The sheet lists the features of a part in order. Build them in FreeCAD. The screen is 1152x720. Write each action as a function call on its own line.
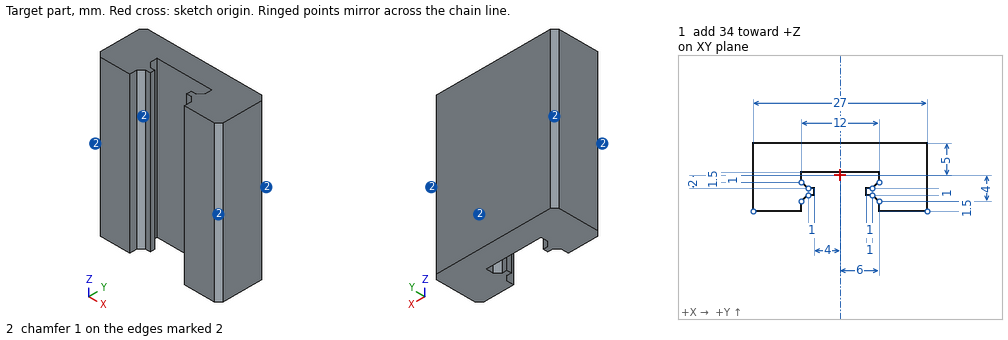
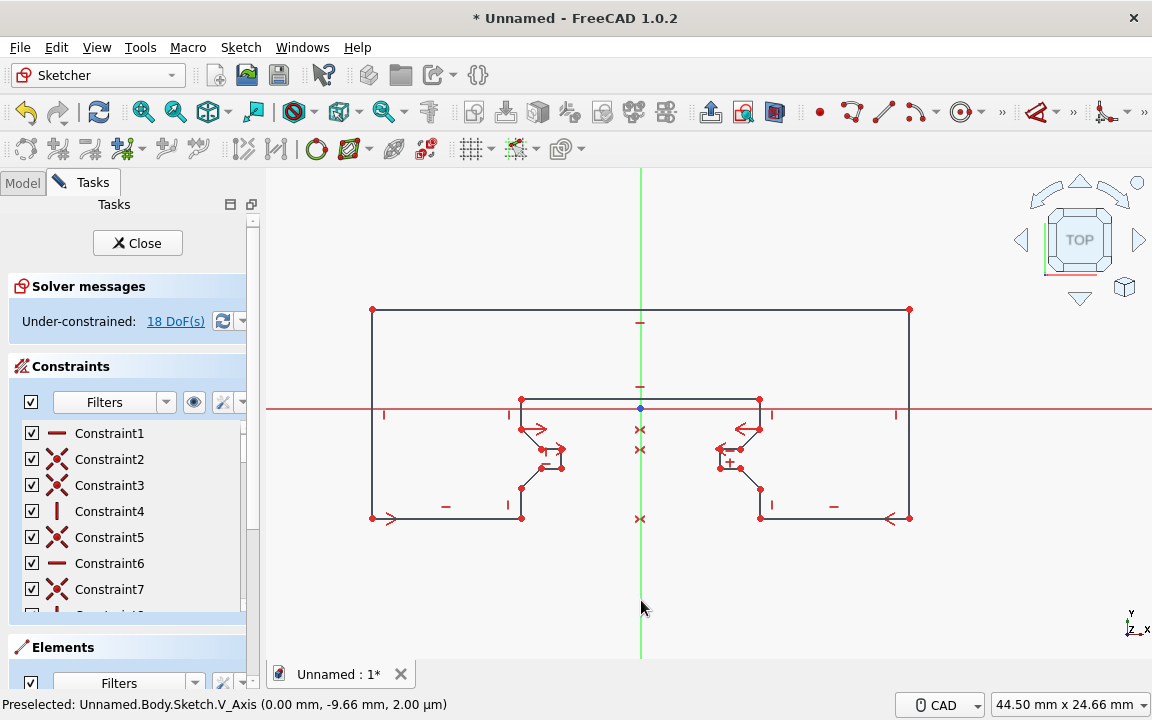
click(760, 489)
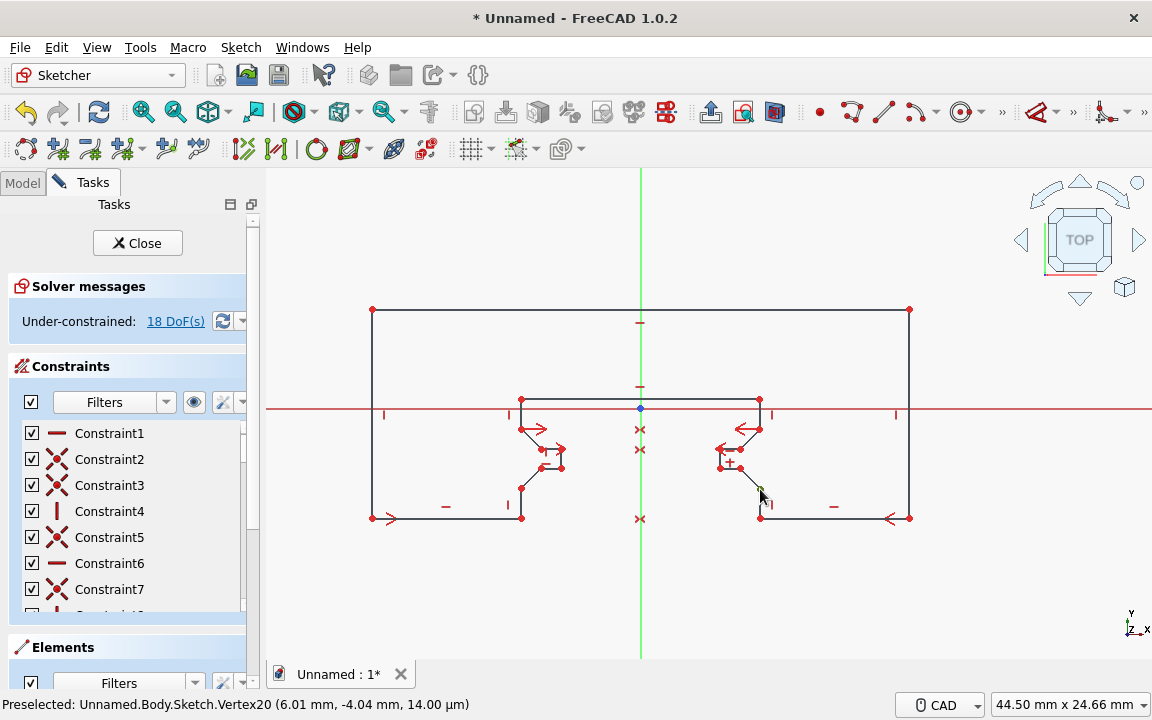
click(521, 489)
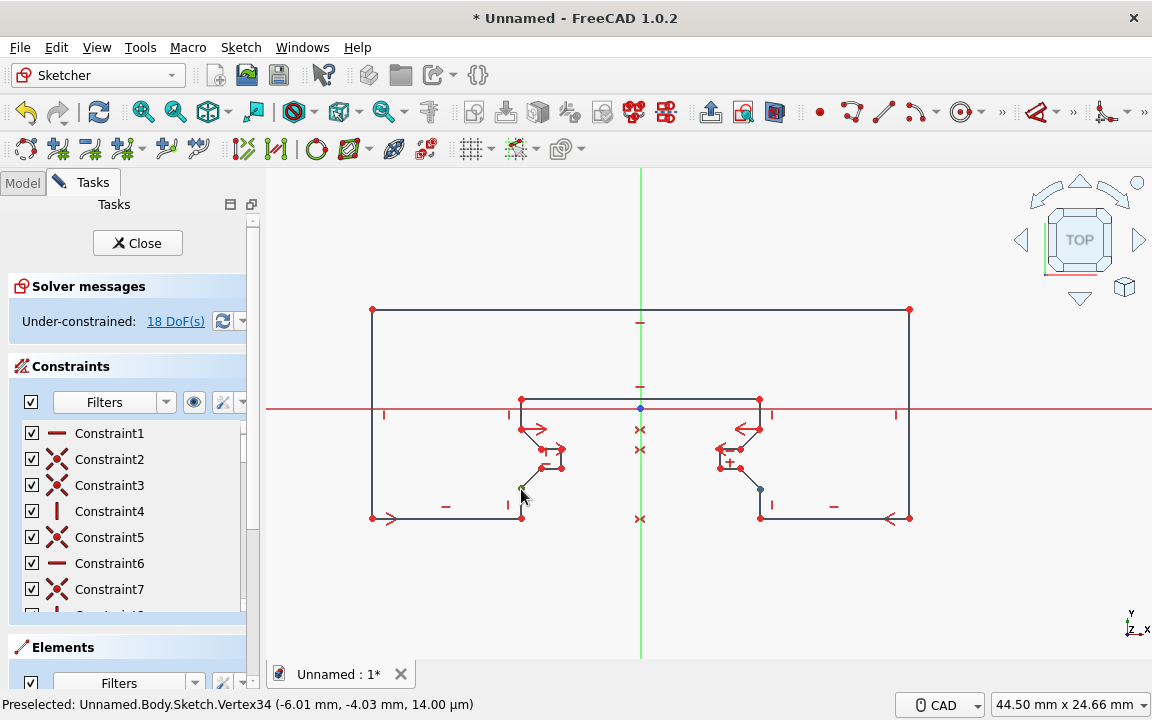
click(641, 600)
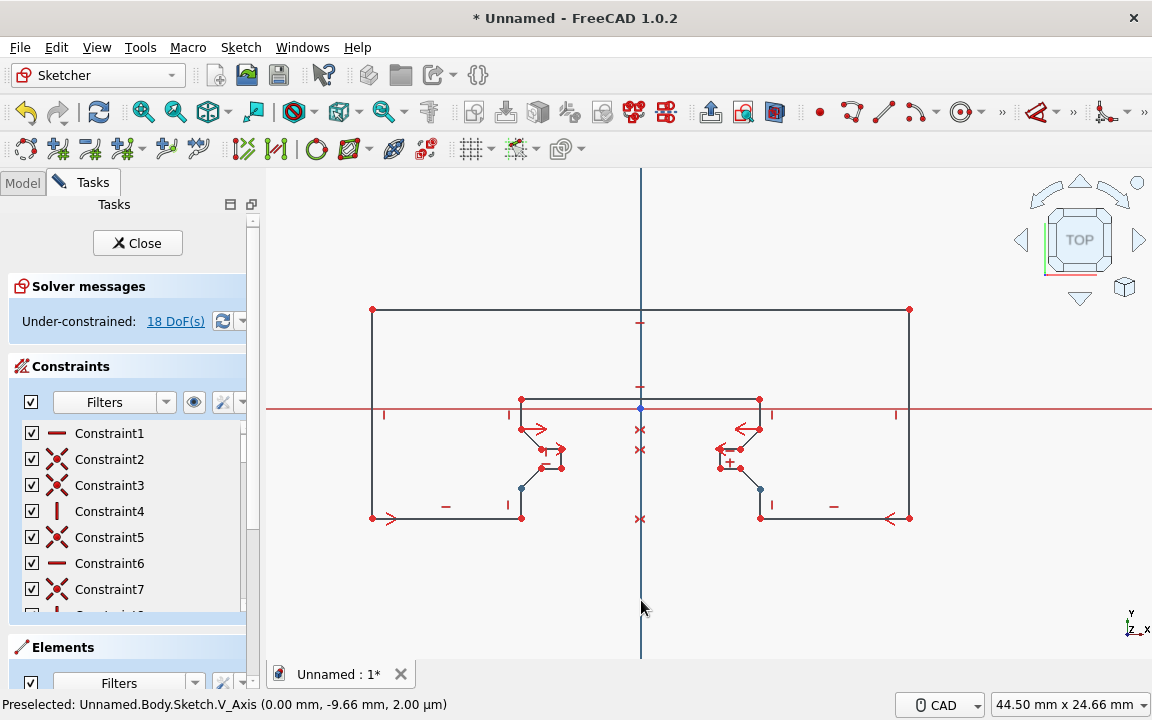
key(s)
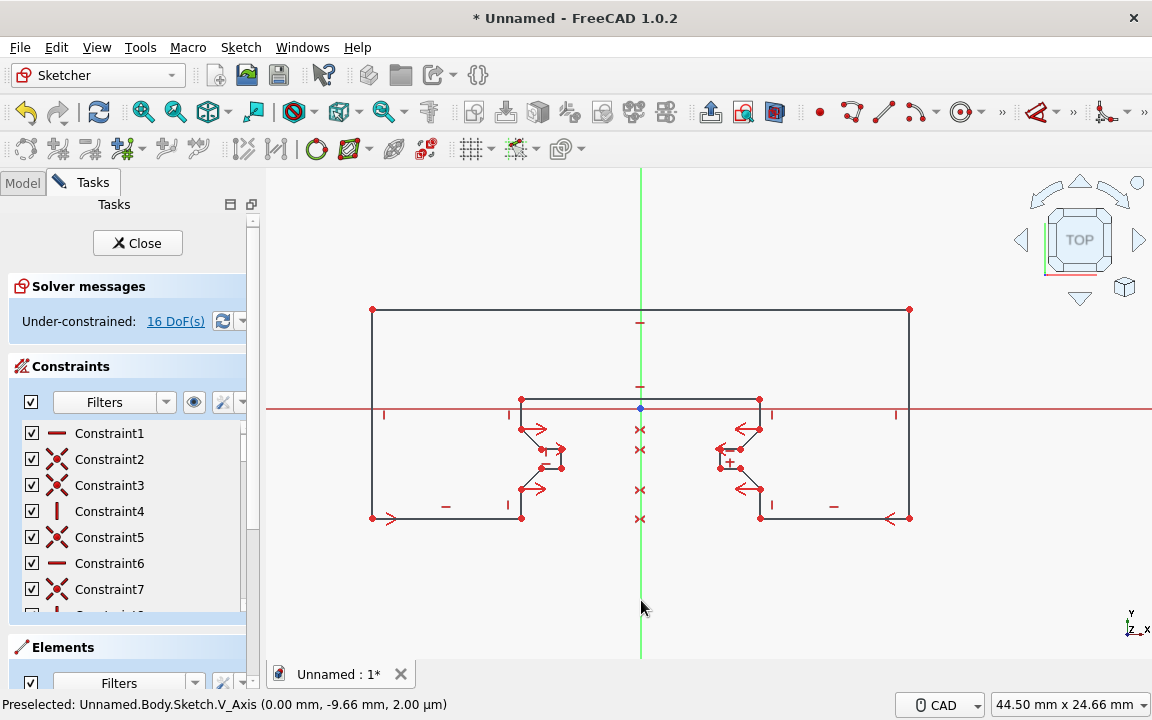
click(740, 469)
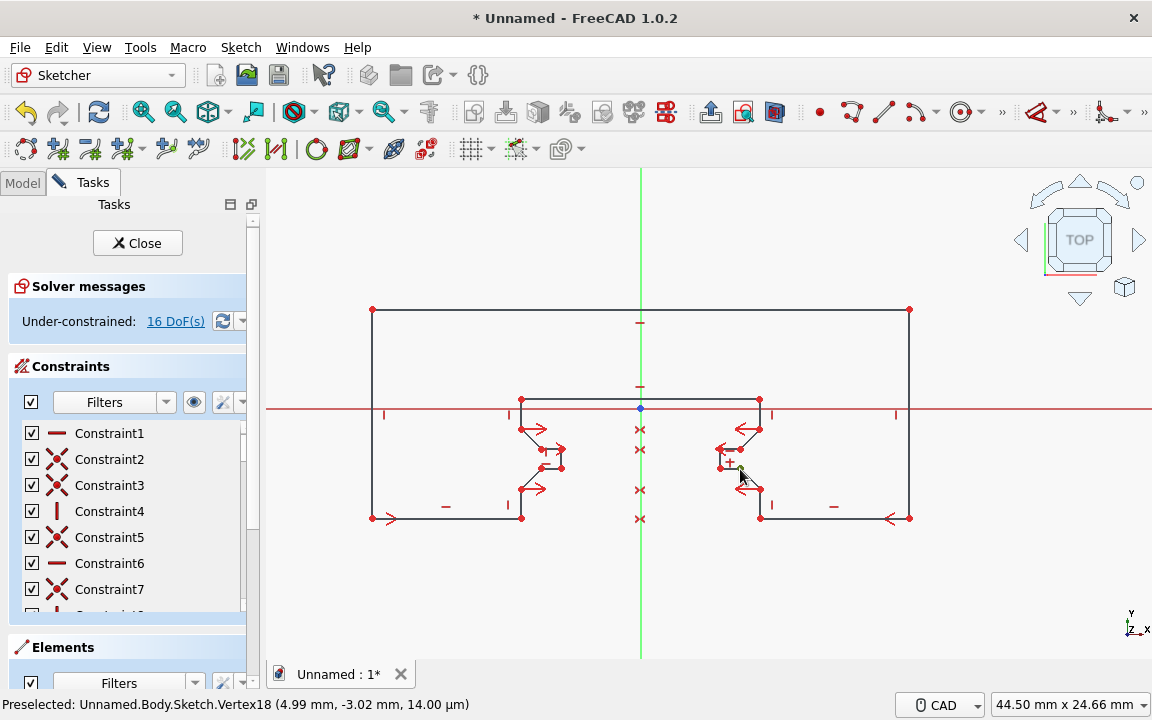
click(541, 469)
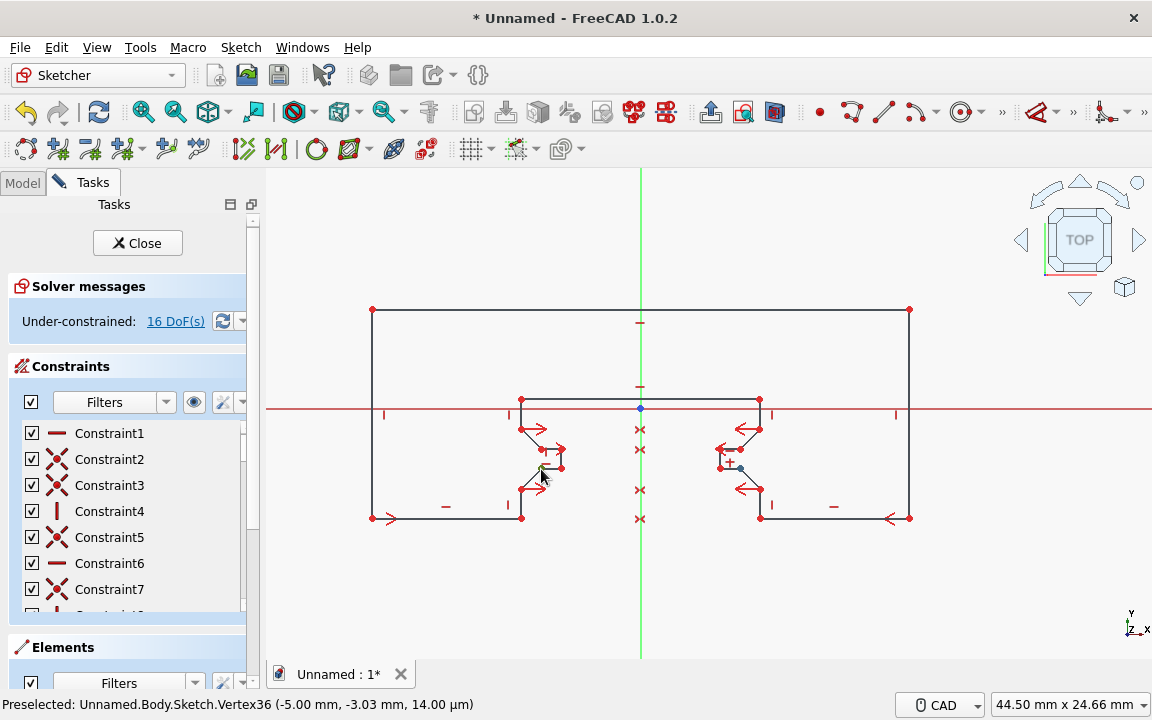
click(641, 600)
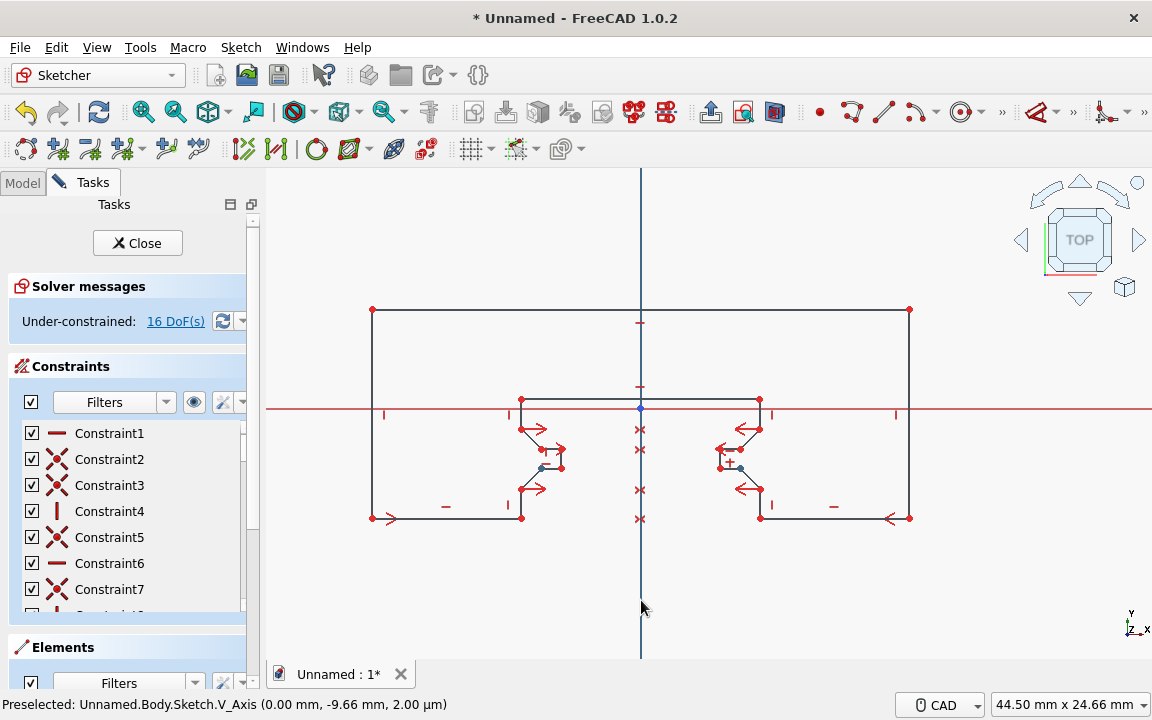
key(s)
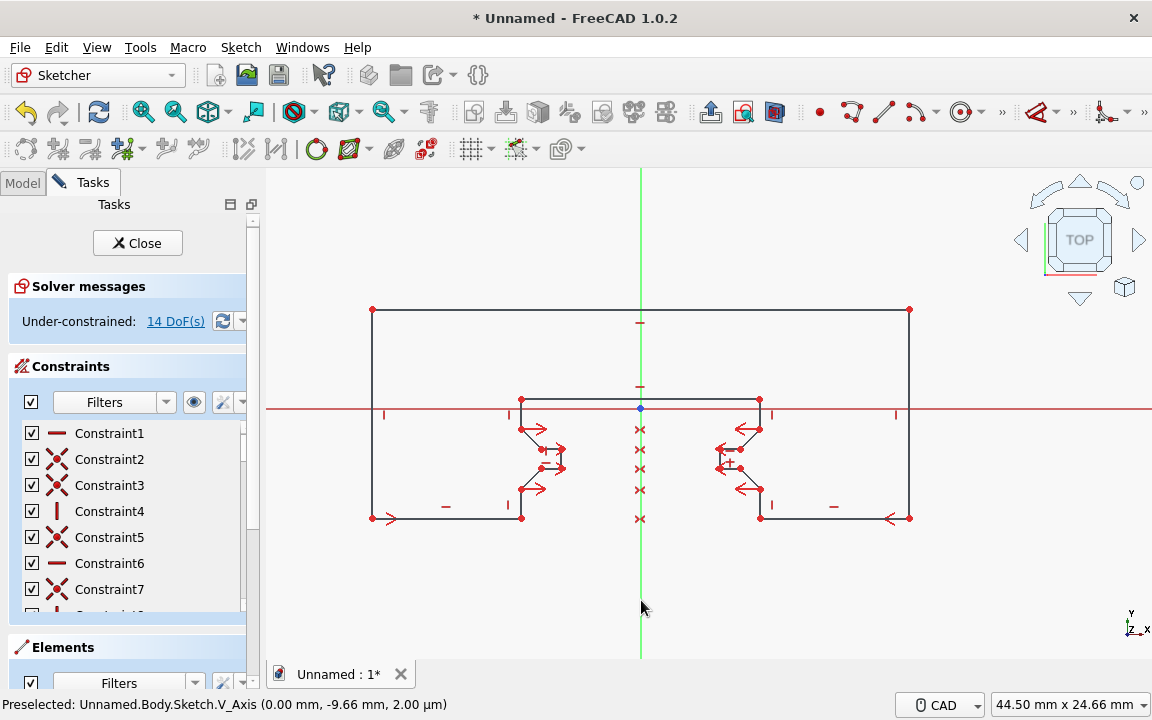
click(1036, 112)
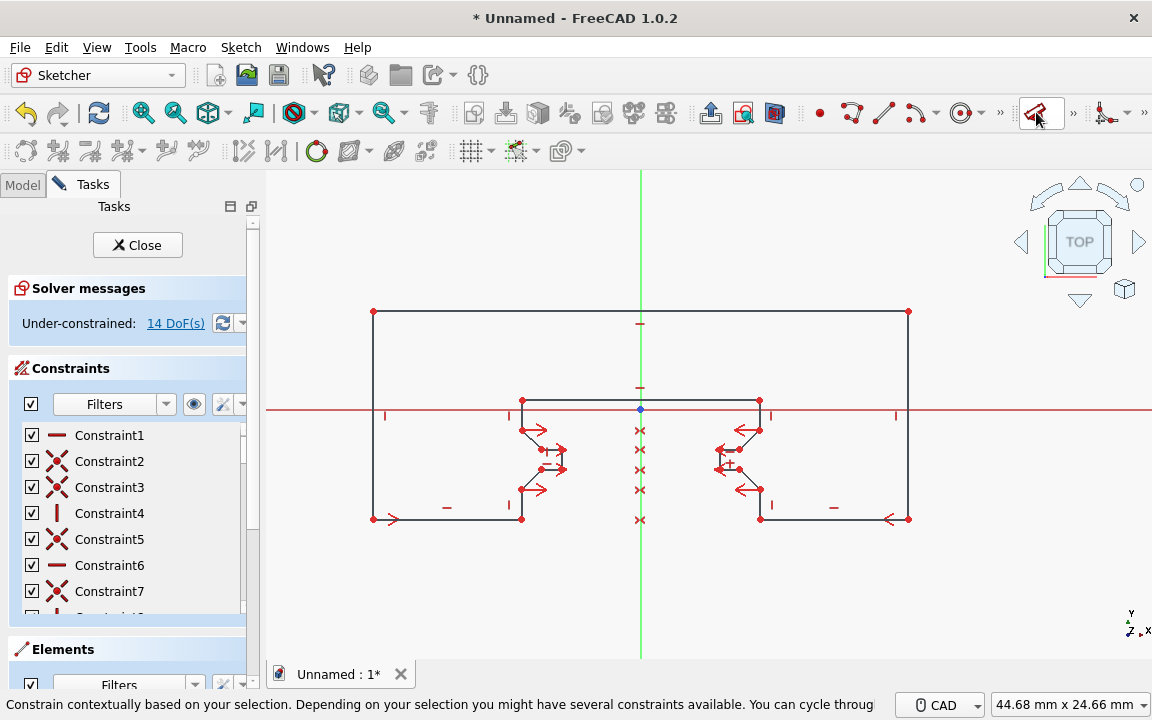
scroll(552, 450, up, 4)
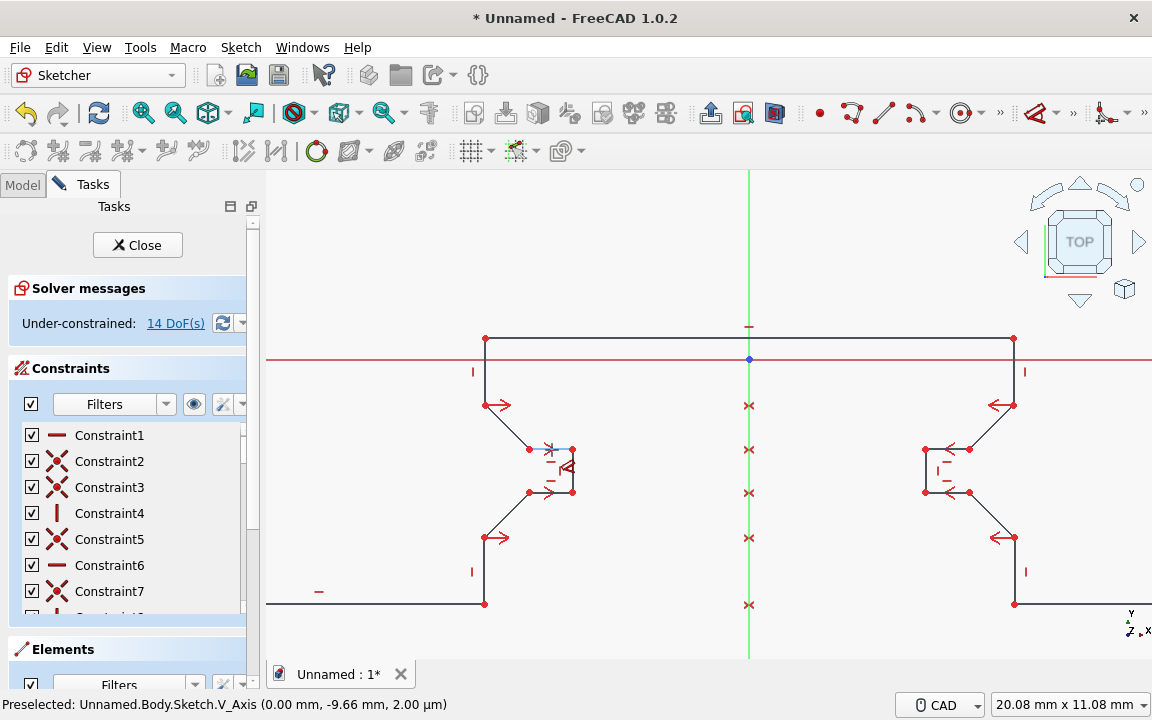
click(551, 449)
click(551, 415)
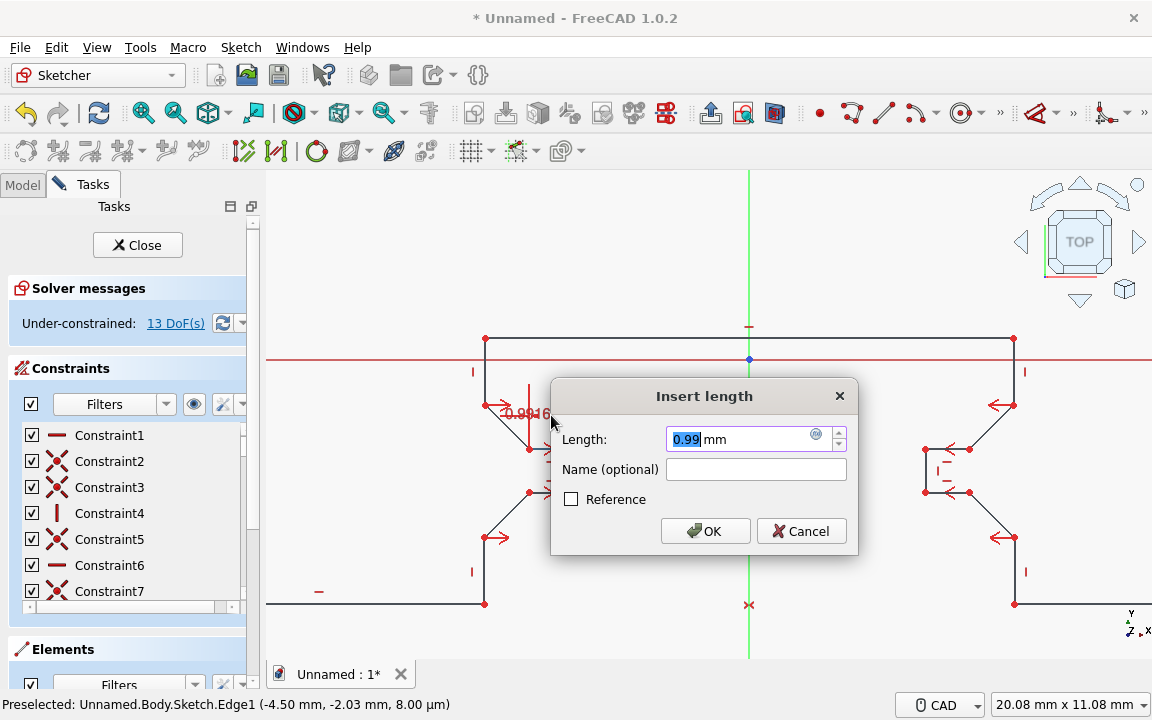
text(1)
key(Return)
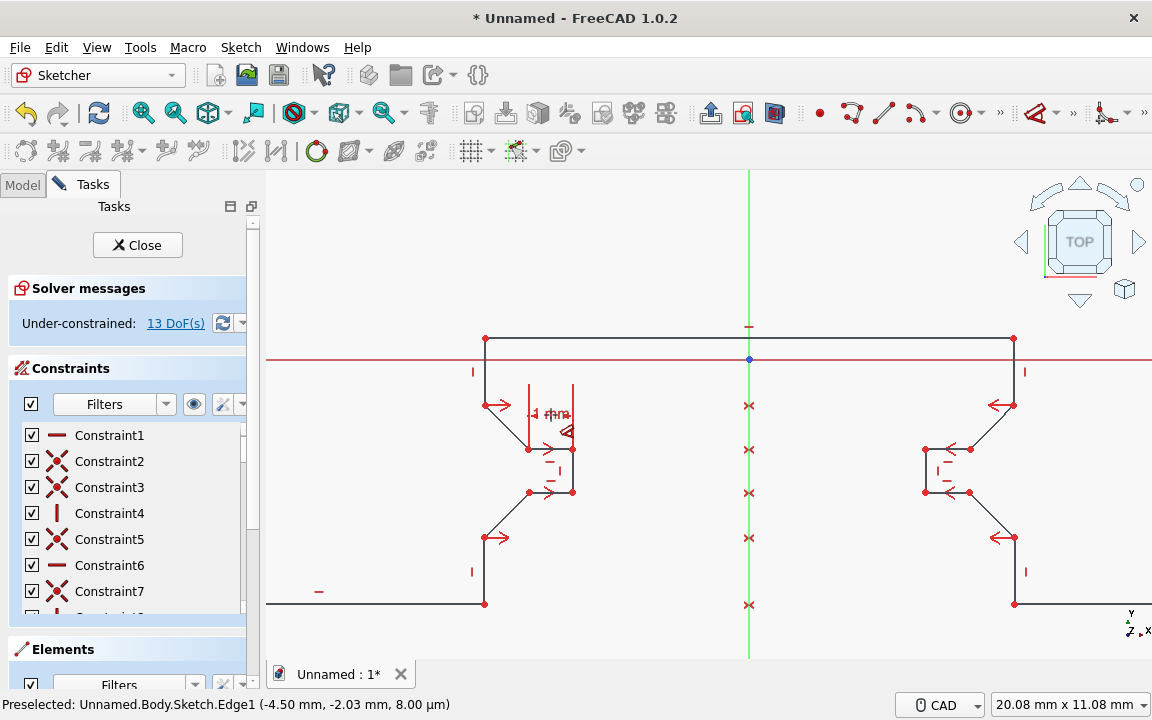
click(957, 449)
click(948, 415)